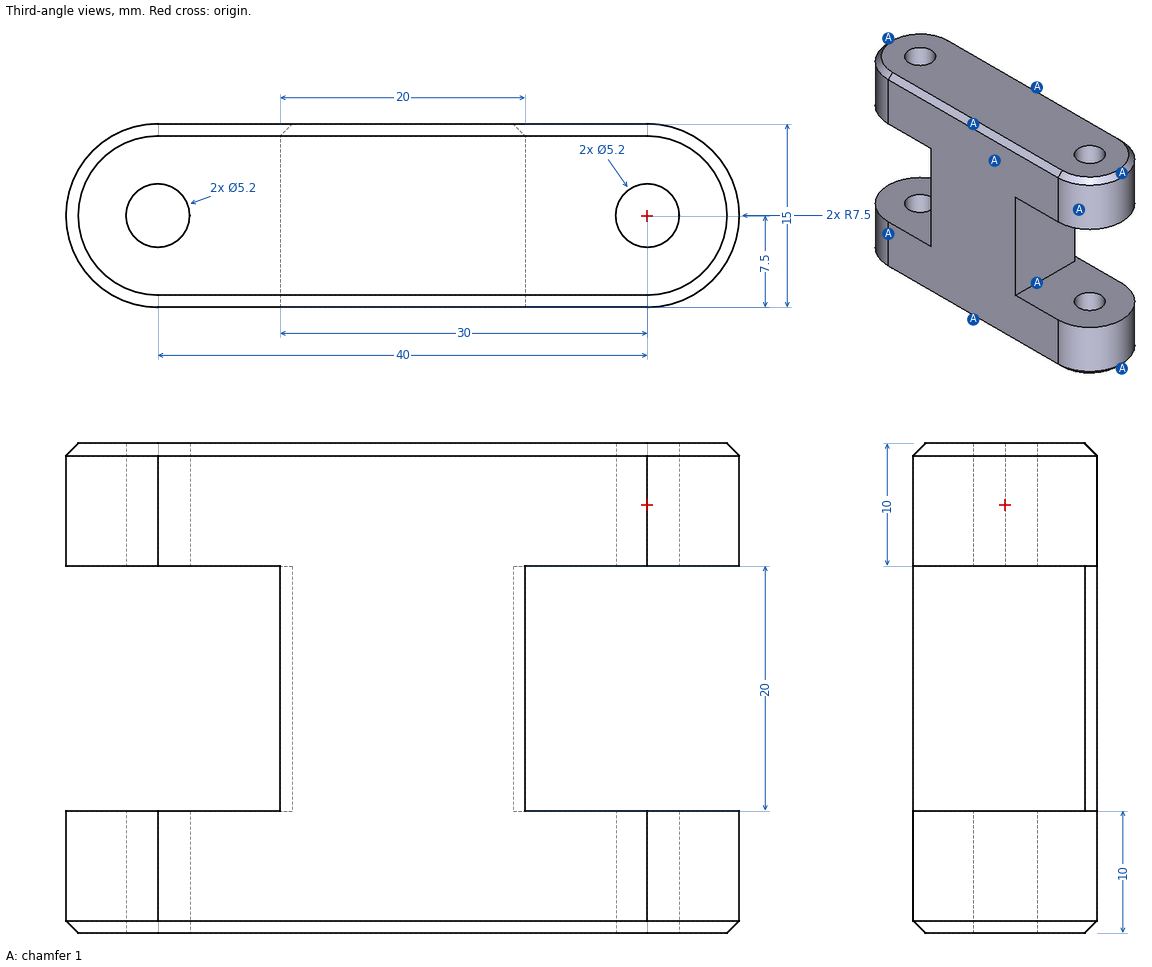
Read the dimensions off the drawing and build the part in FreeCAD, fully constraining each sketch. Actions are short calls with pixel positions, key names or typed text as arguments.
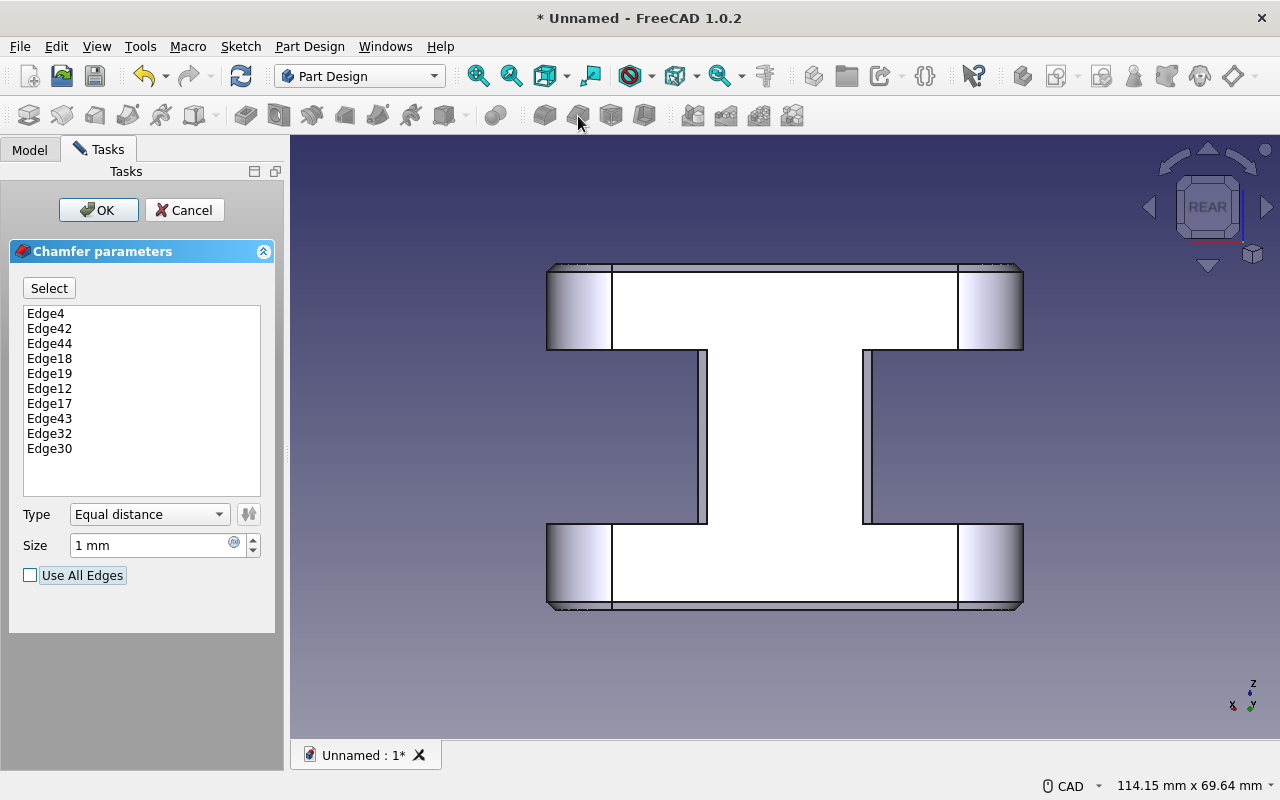
click(99, 210)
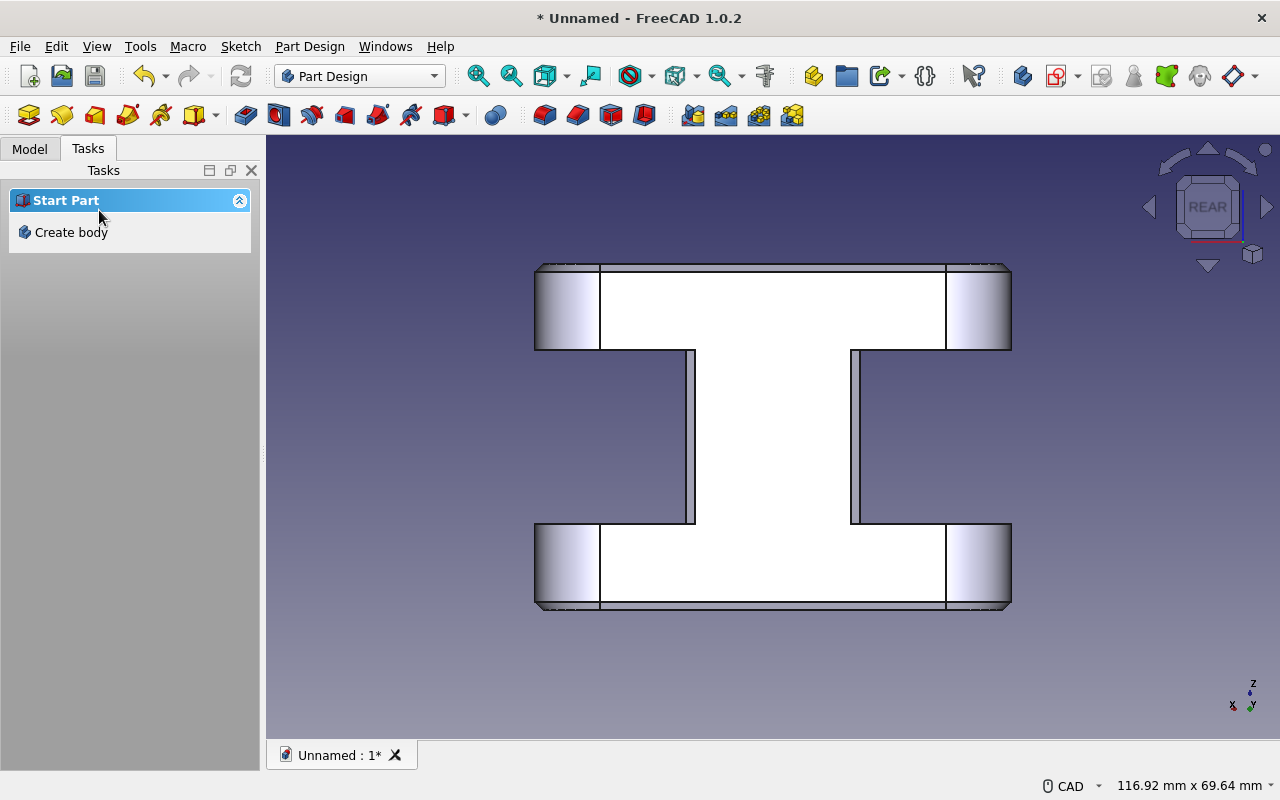
key(0)